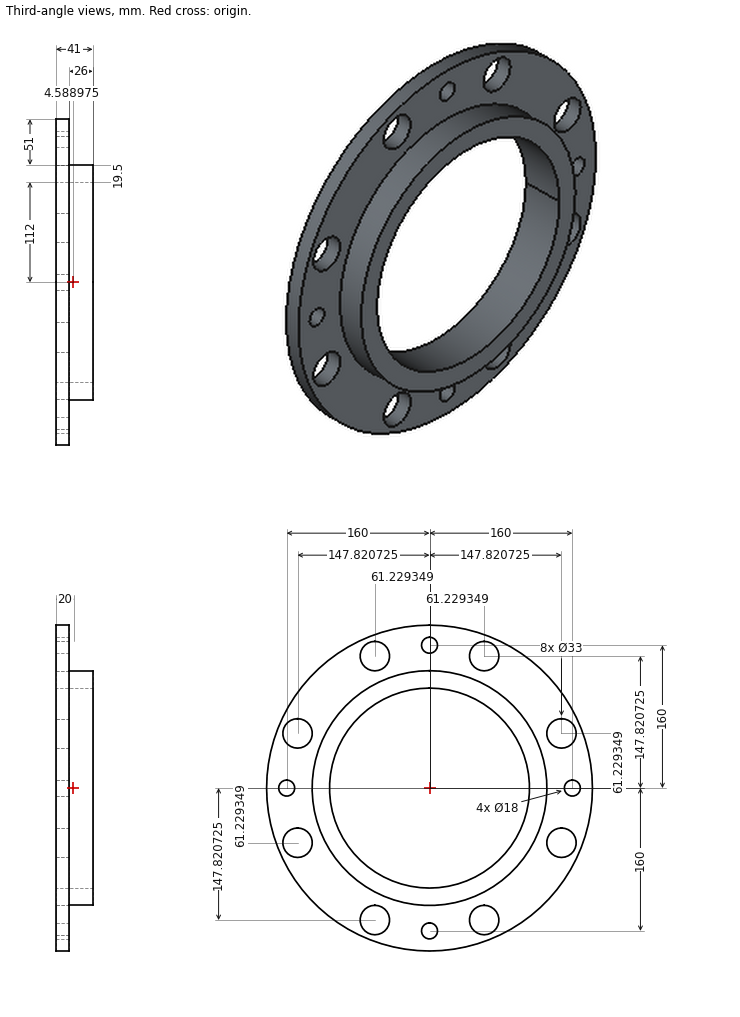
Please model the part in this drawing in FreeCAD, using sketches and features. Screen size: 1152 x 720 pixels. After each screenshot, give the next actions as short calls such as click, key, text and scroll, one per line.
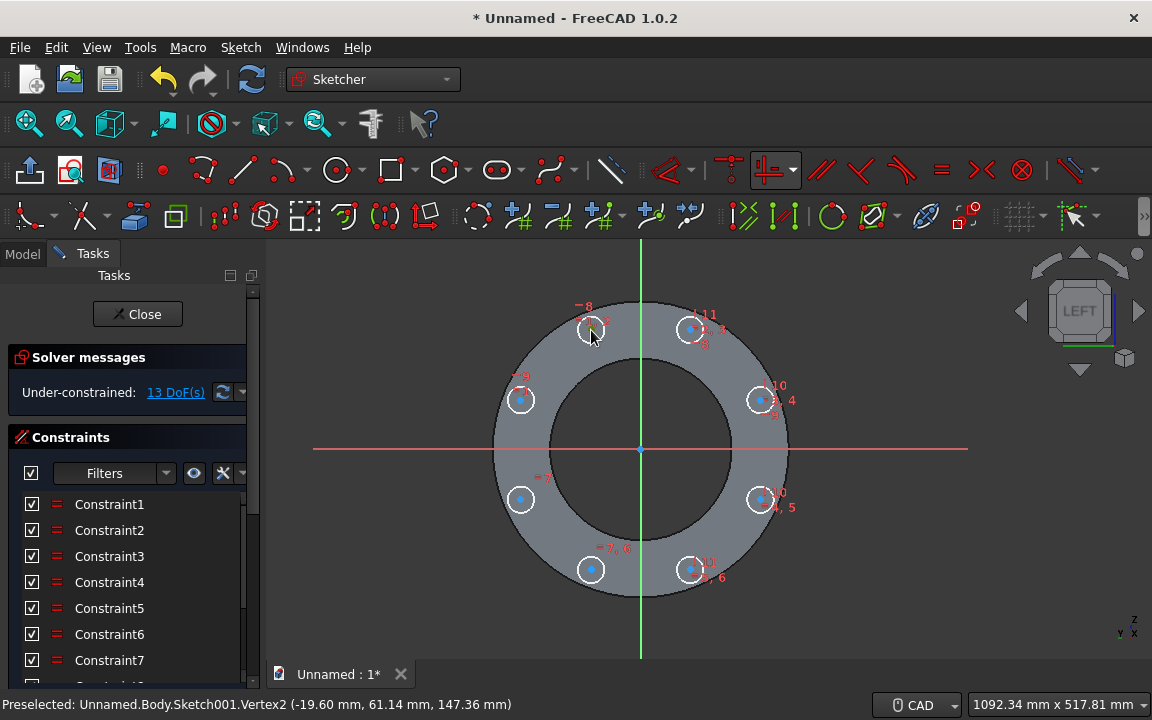
click(591, 570)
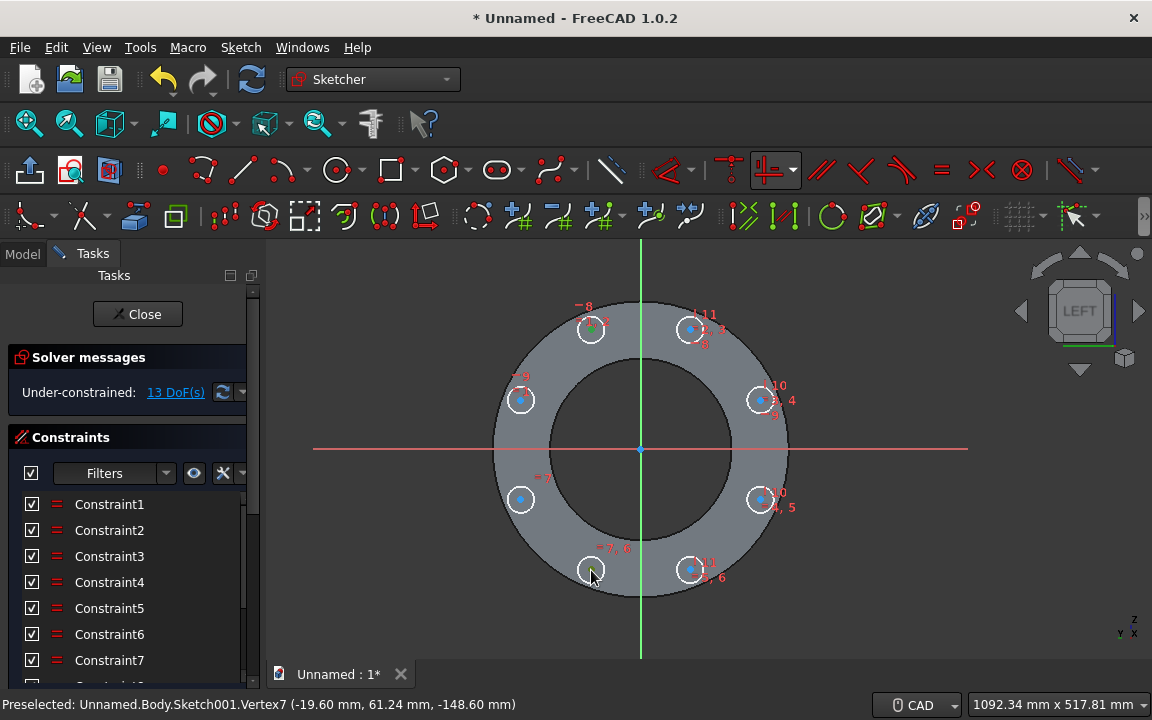
click(796, 170)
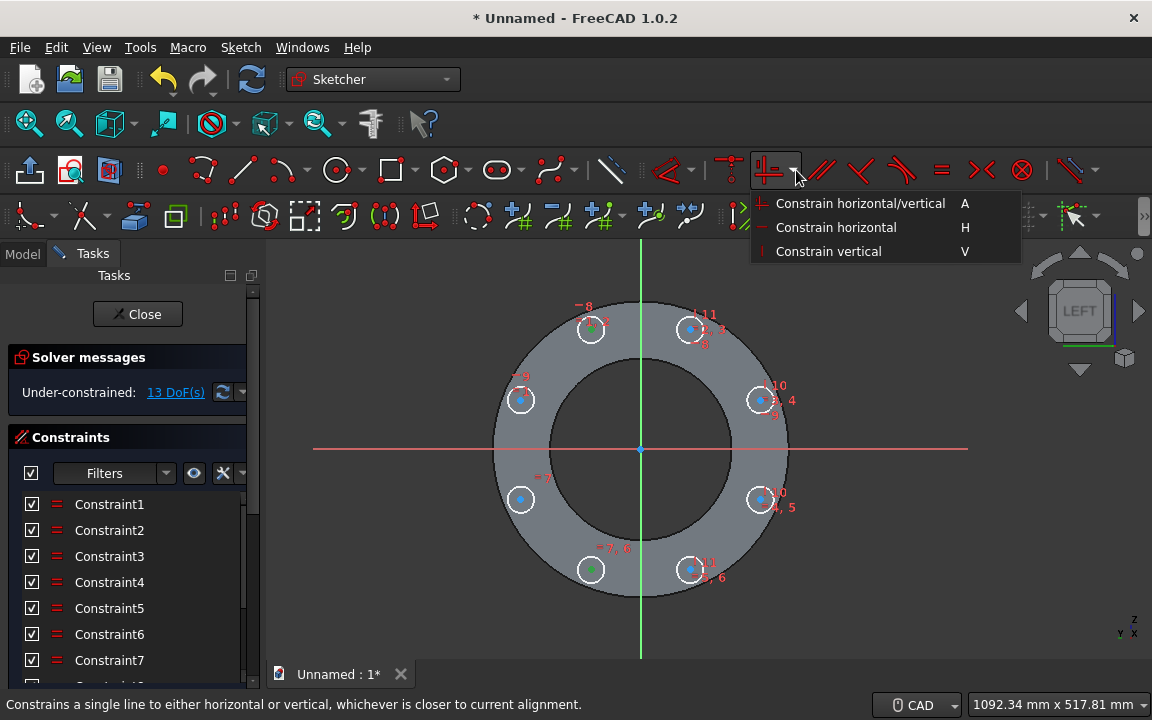
click(886, 251)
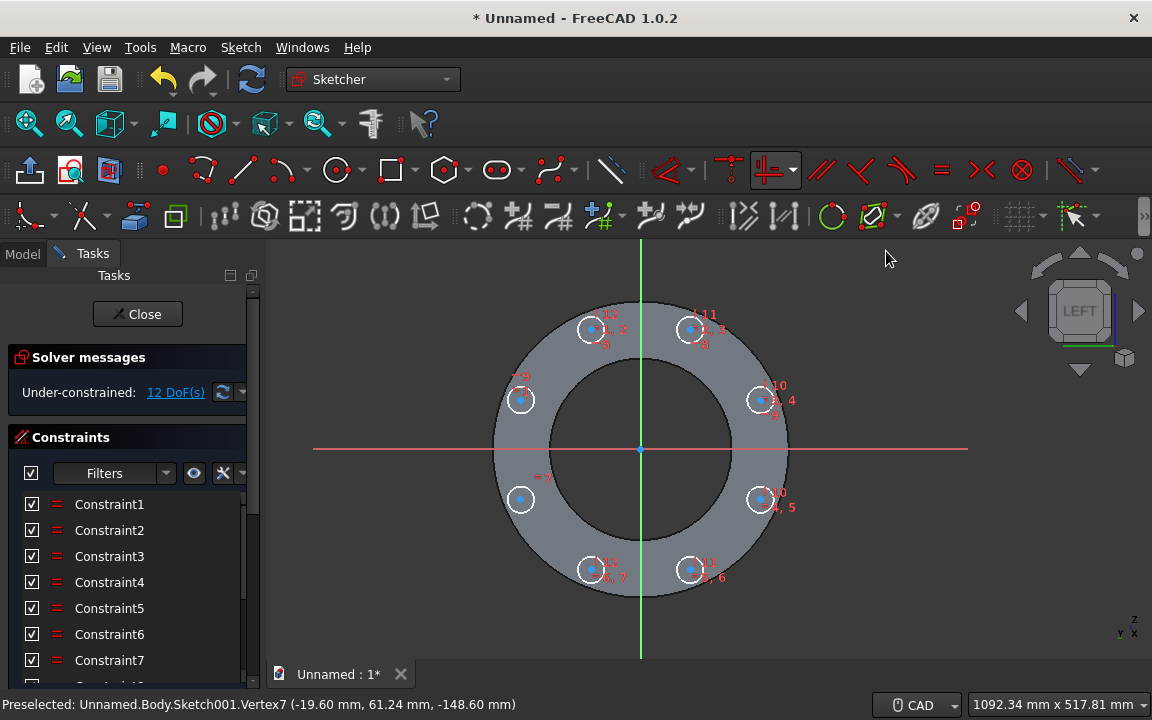
click(688, 572)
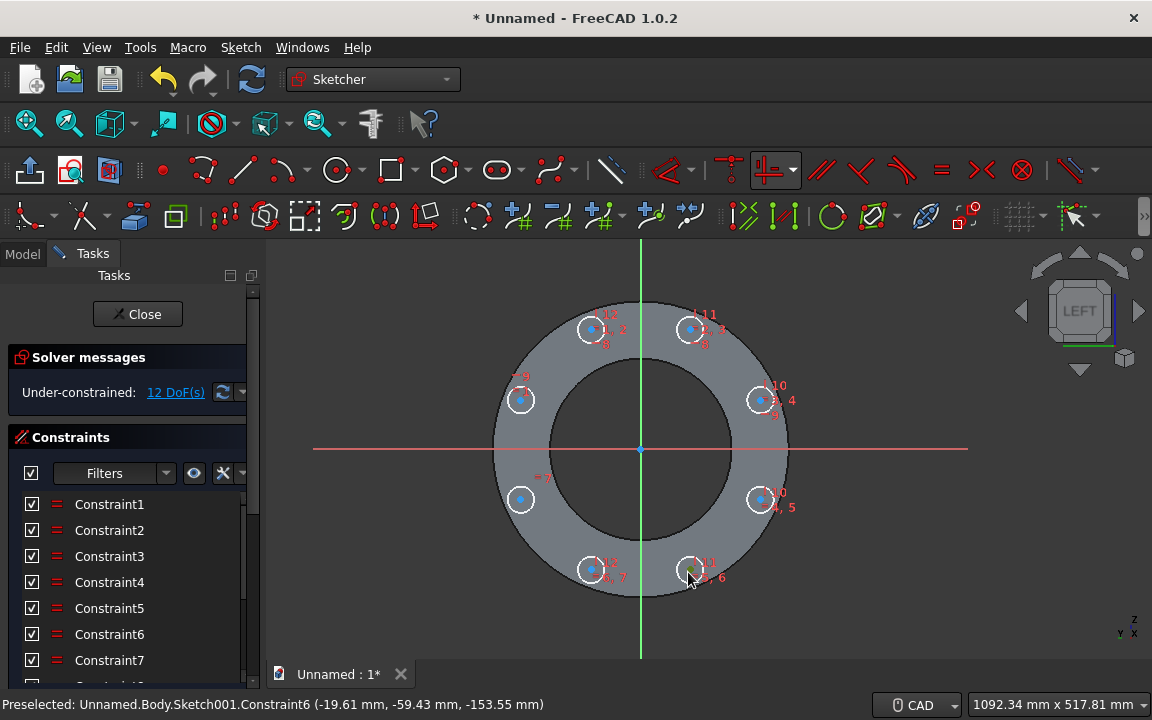
click(589, 572)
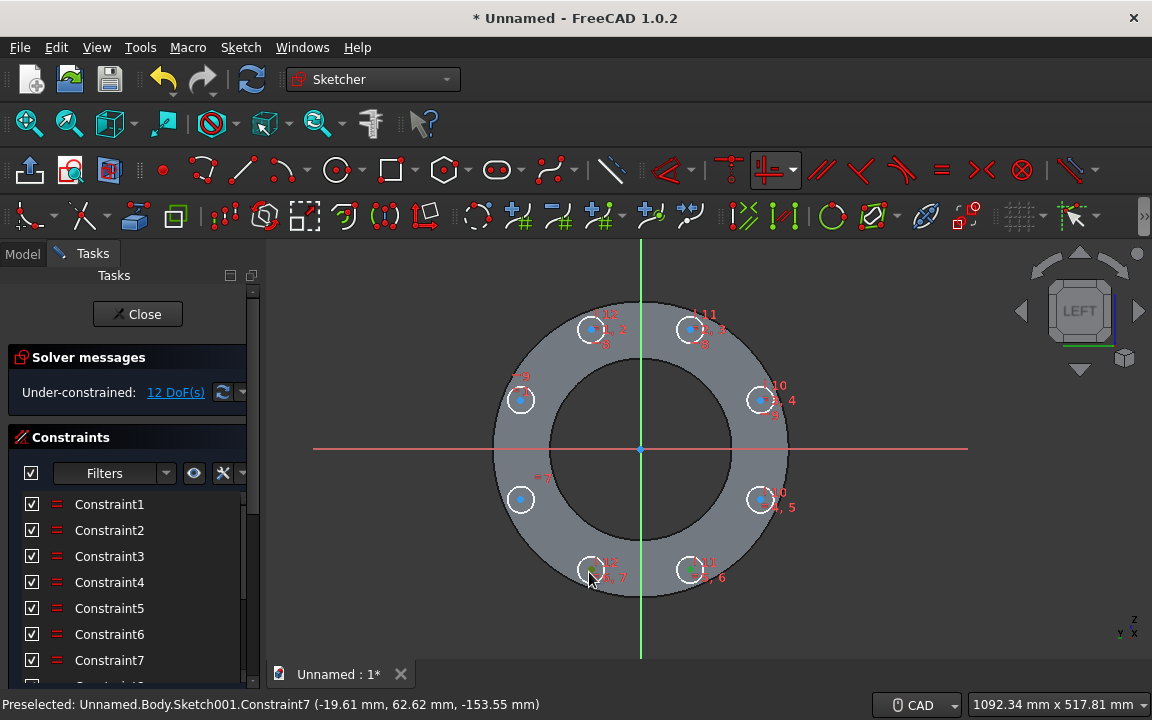
click(796, 170)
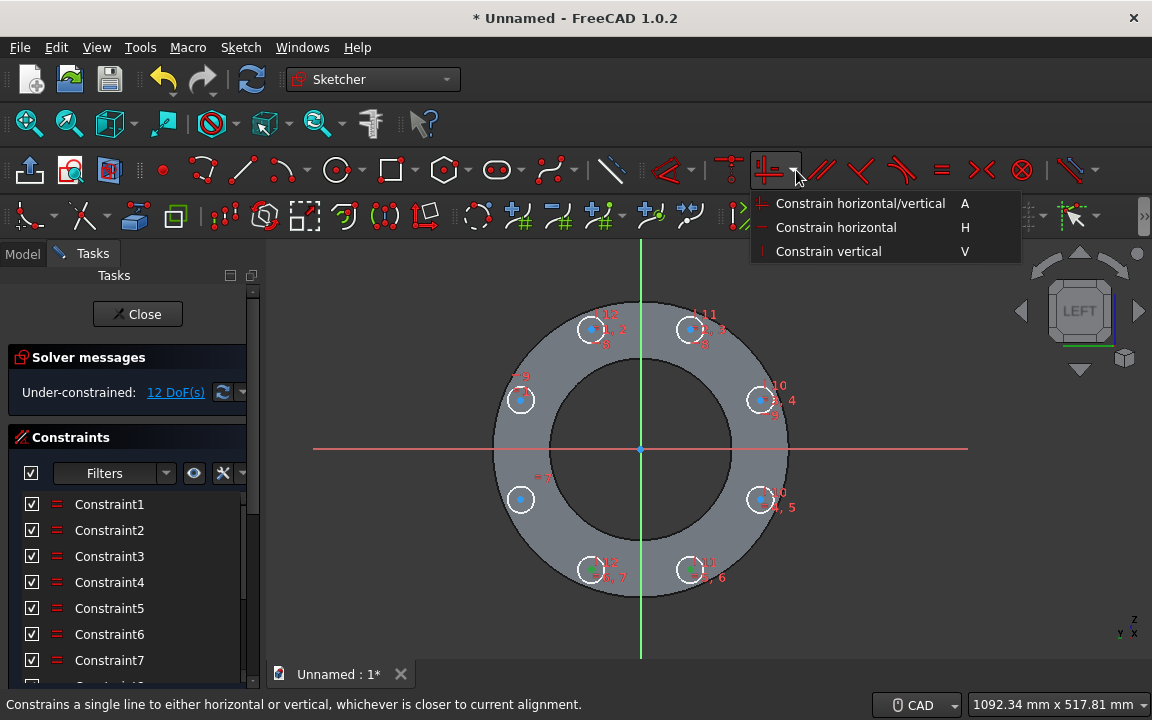
click(886, 227)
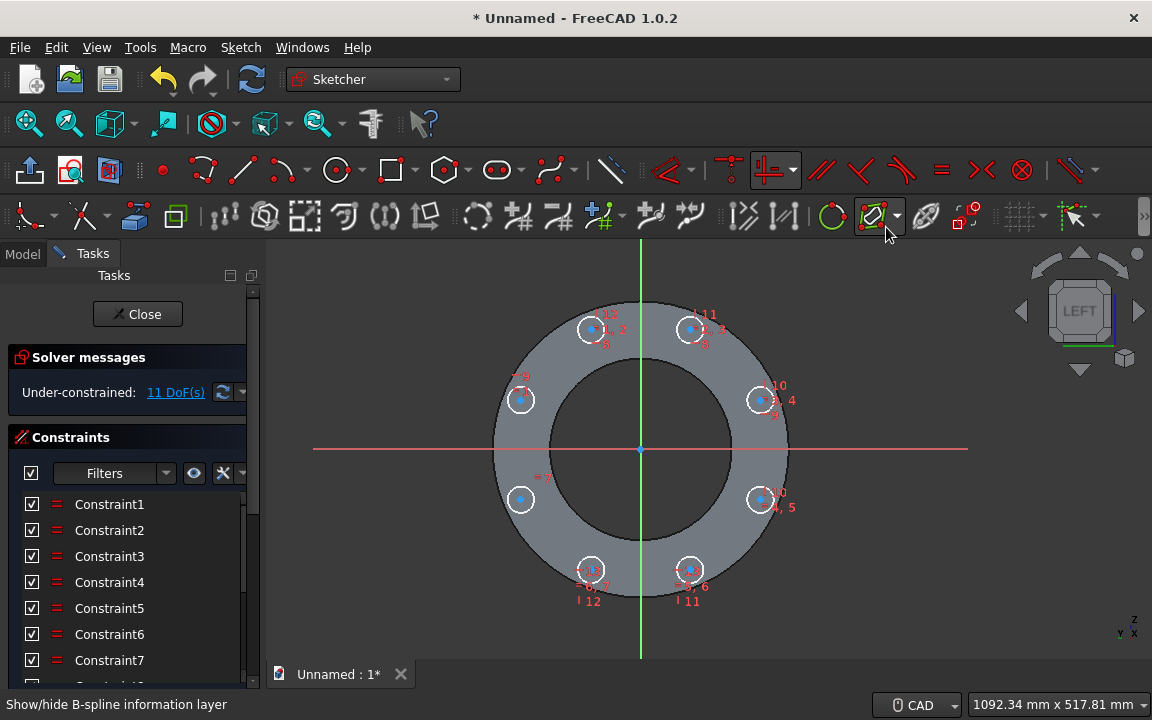
click(521, 400)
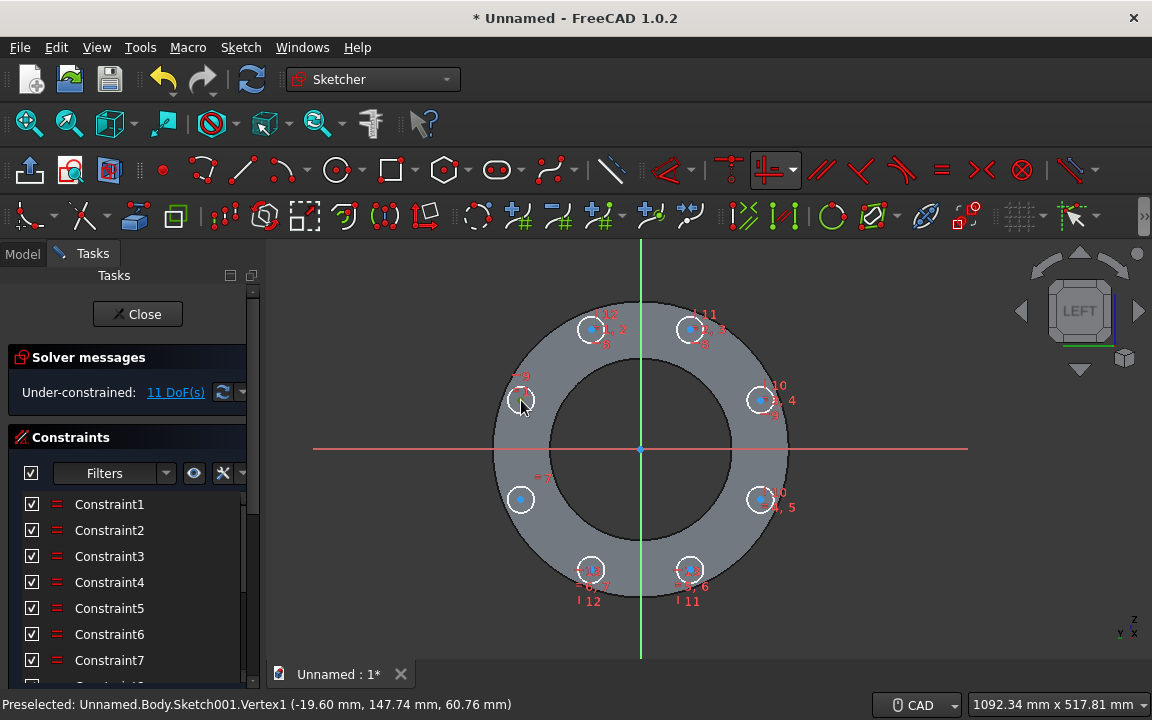
click(521, 500)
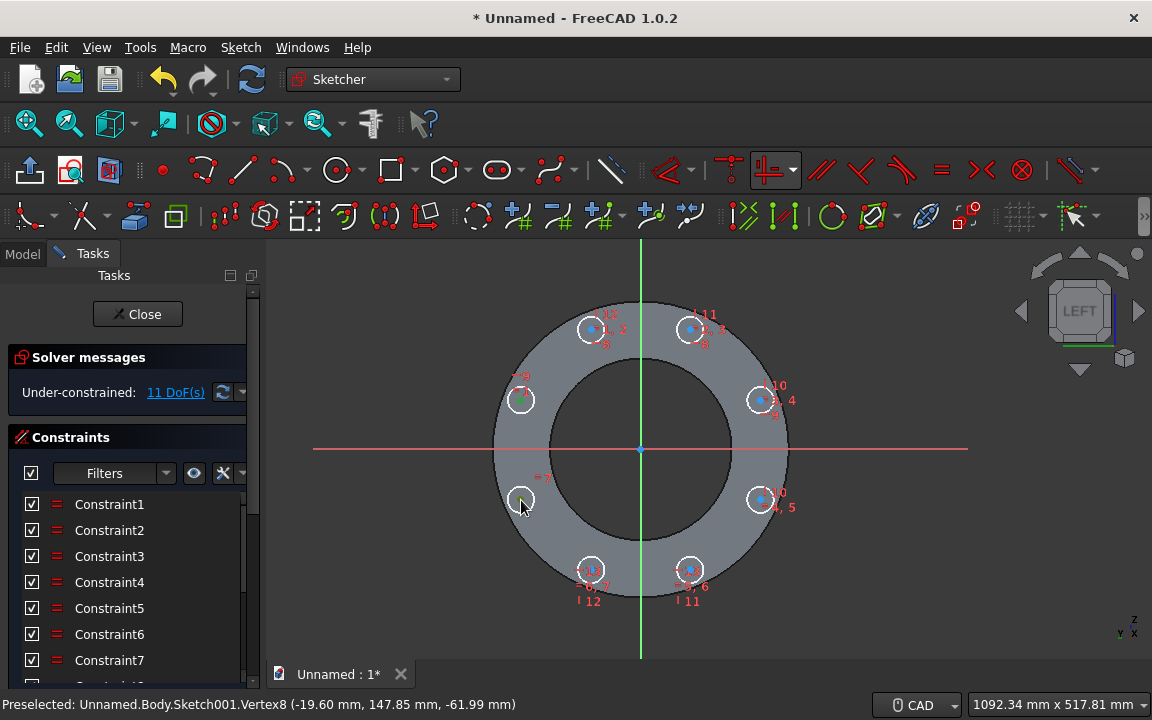
click(796, 170)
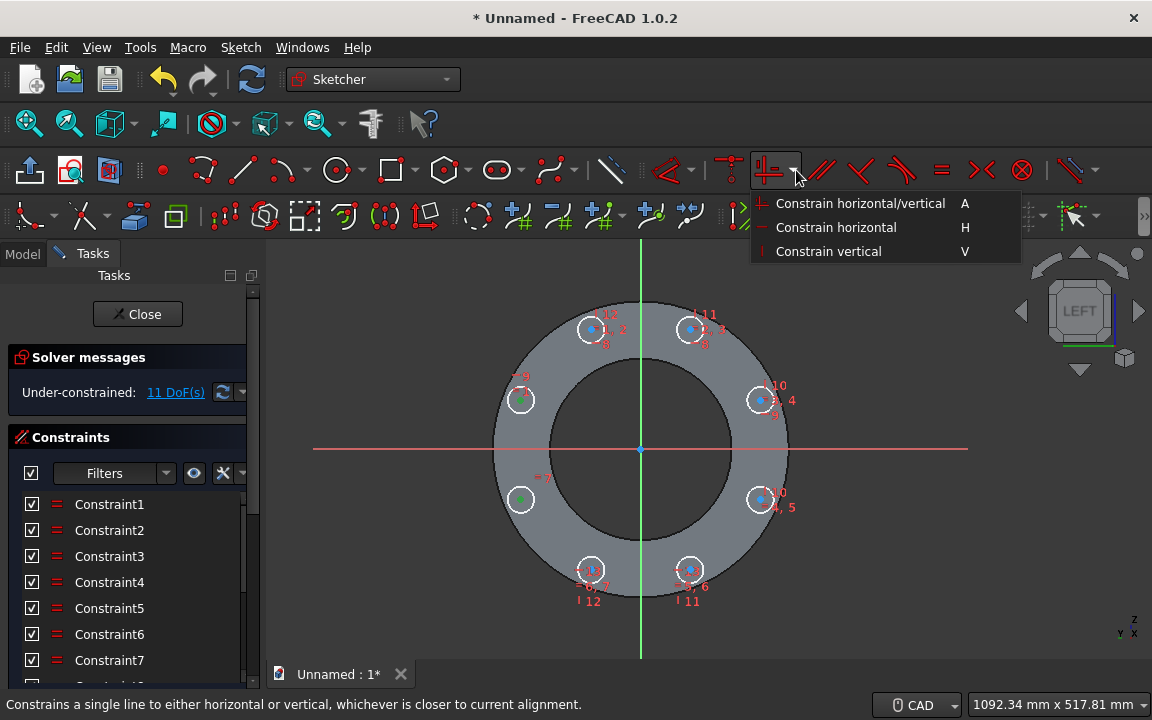
click(886, 251)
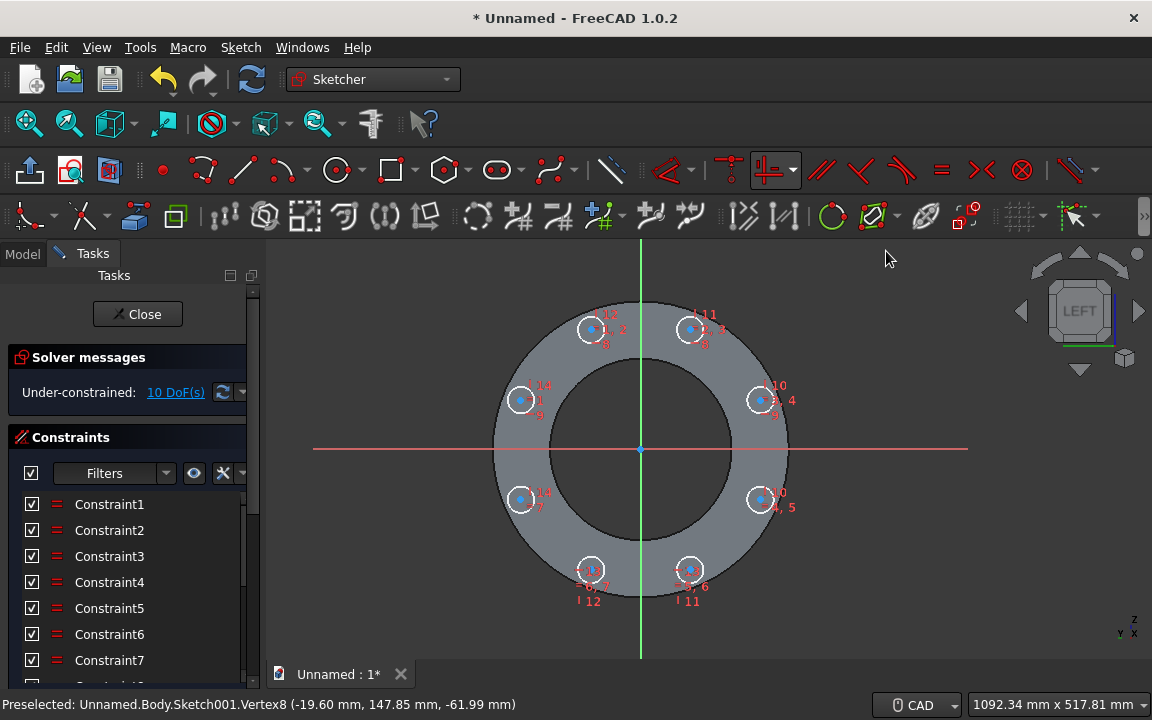
click(758, 502)